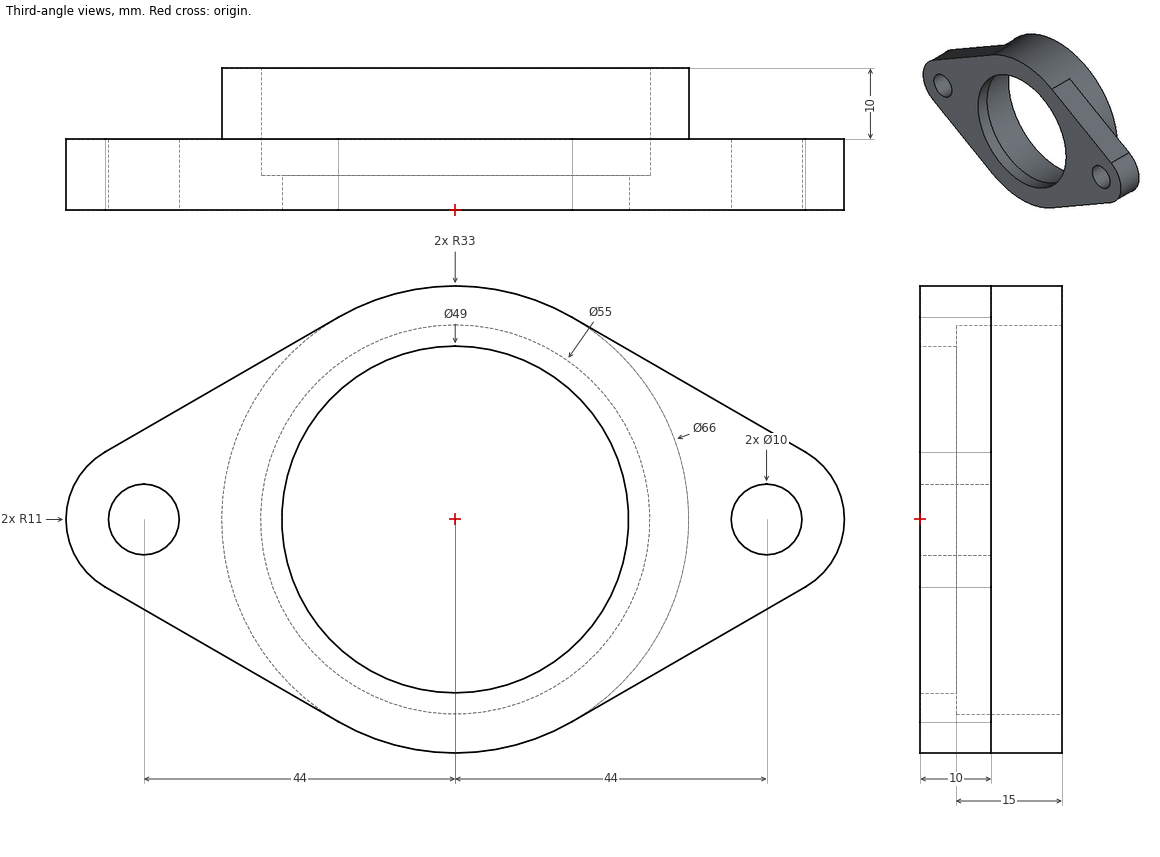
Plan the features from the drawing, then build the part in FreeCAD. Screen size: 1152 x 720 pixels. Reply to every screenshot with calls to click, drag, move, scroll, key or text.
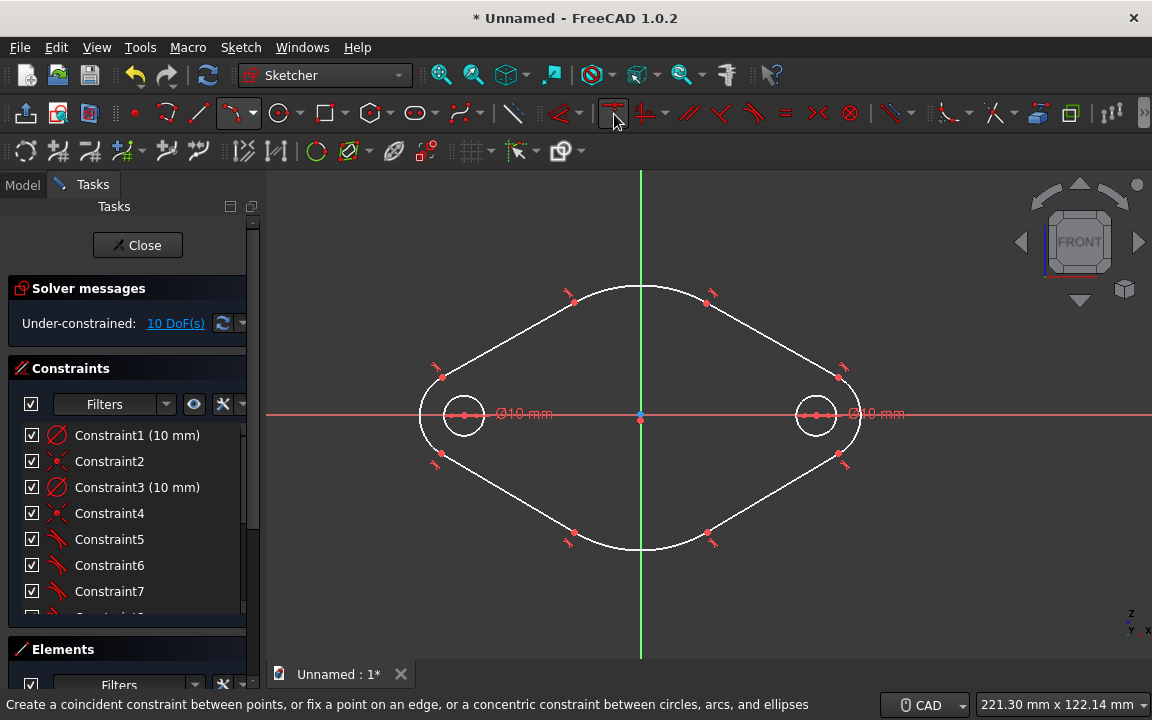
scroll(641, 417, up, 4)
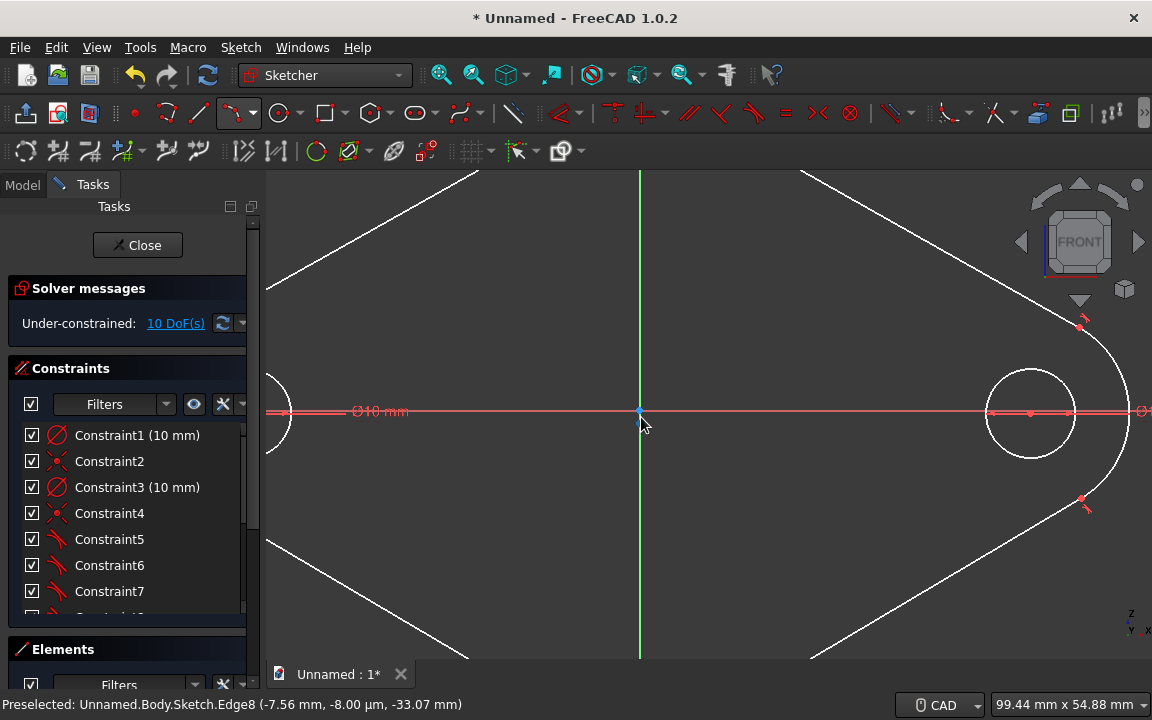
drag(630, 401, 650, 434)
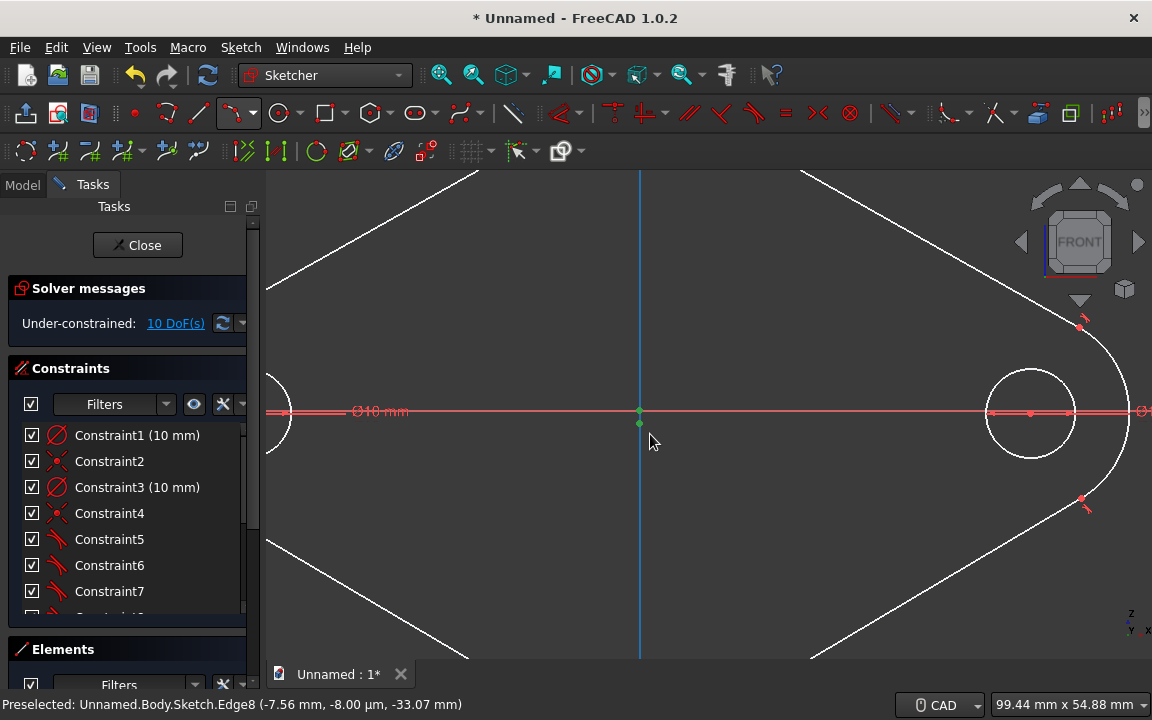
click(614, 114)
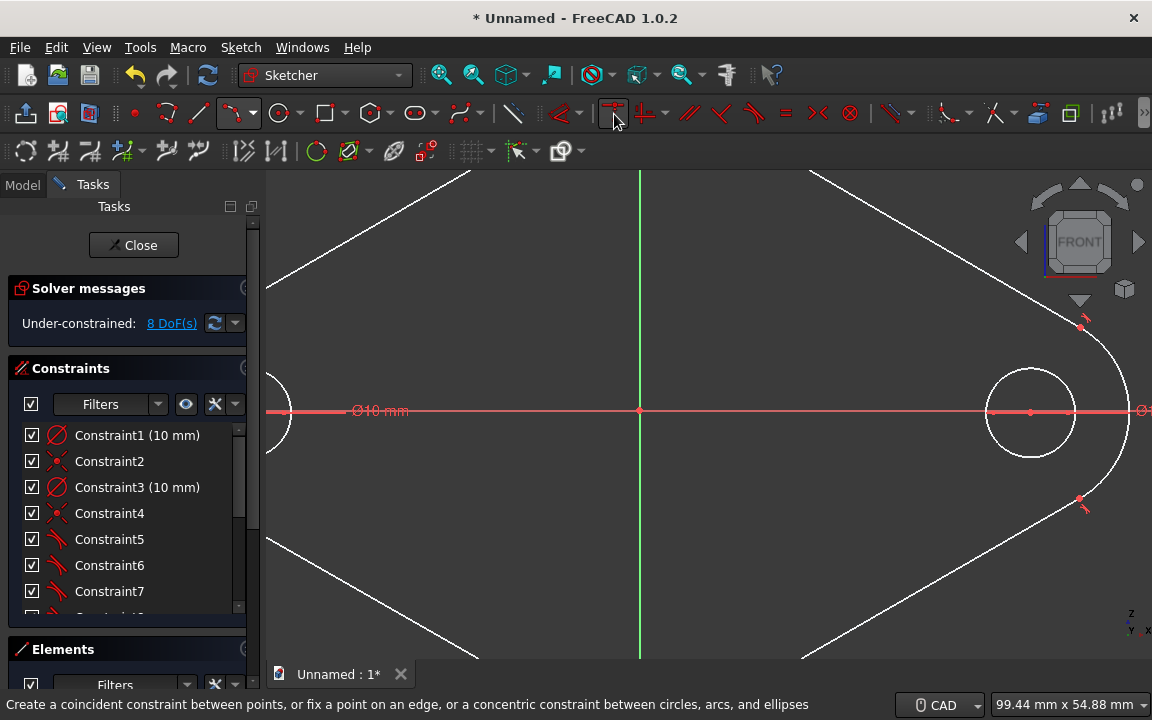
scroll(641, 419, down, 3)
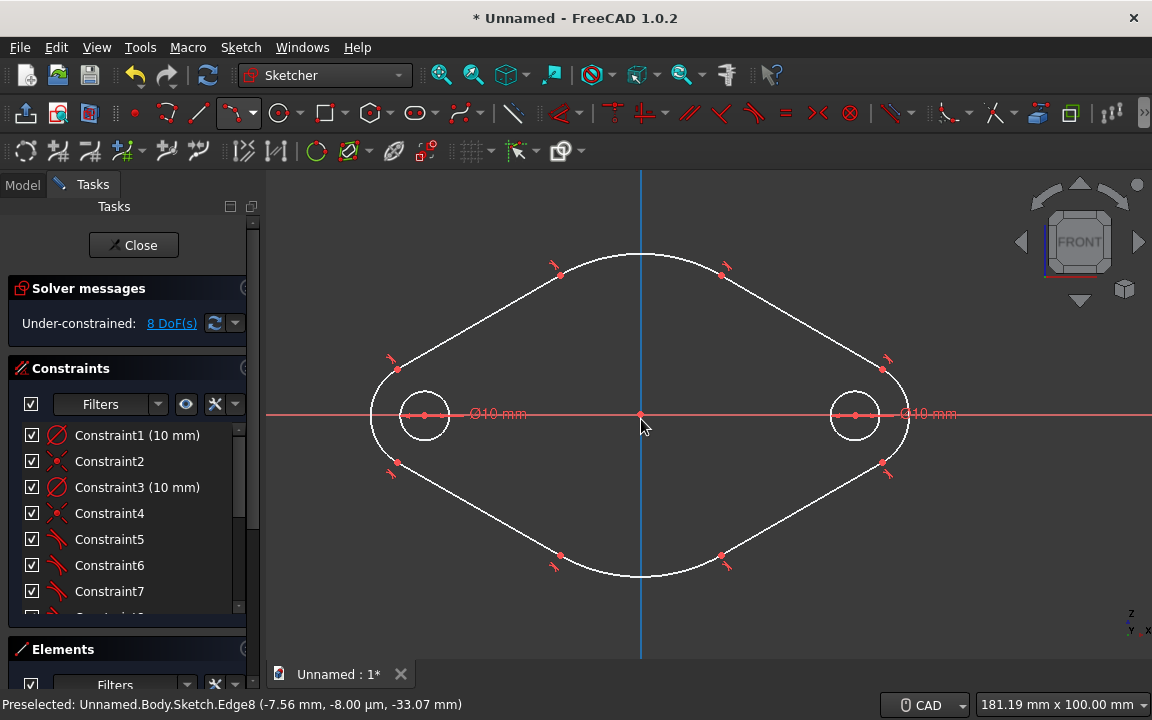
click(375, 394)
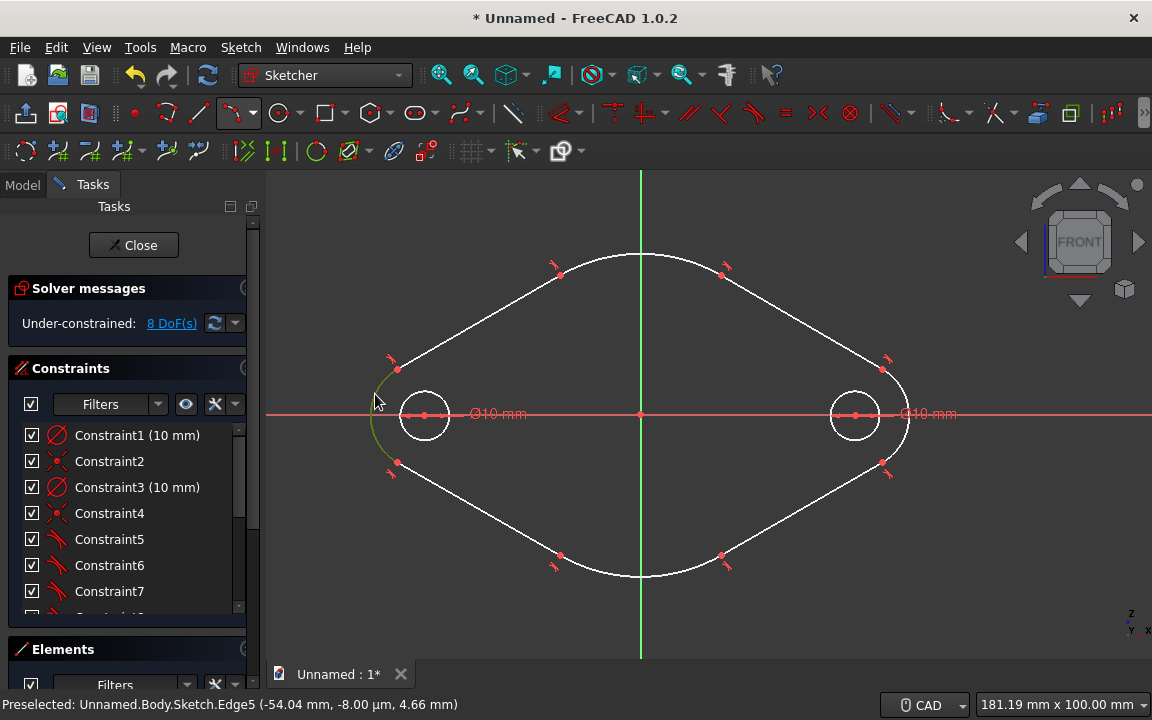
click(904, 438)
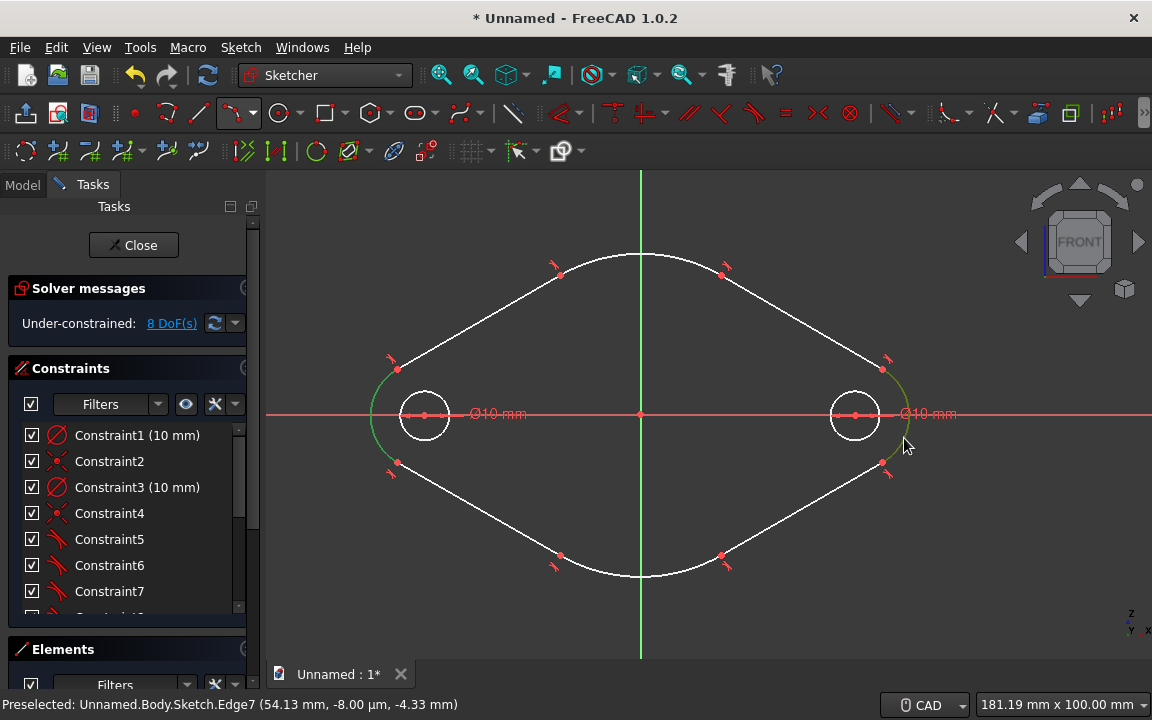
click(786, 114)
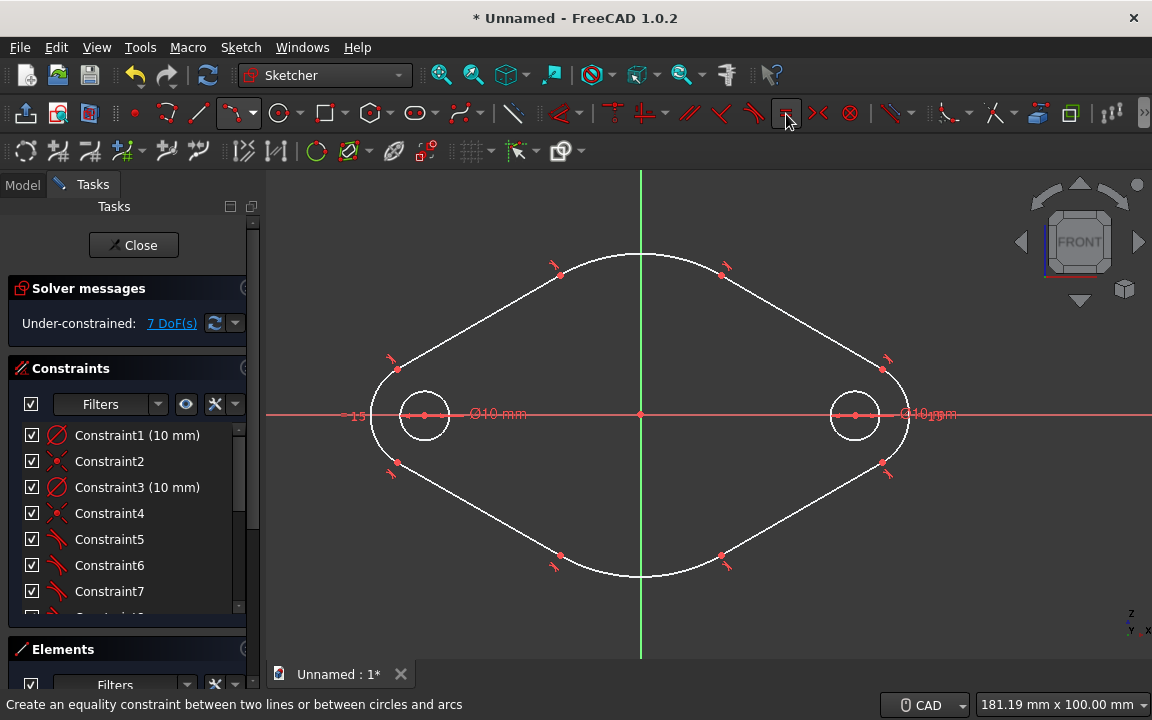
click(674, 257)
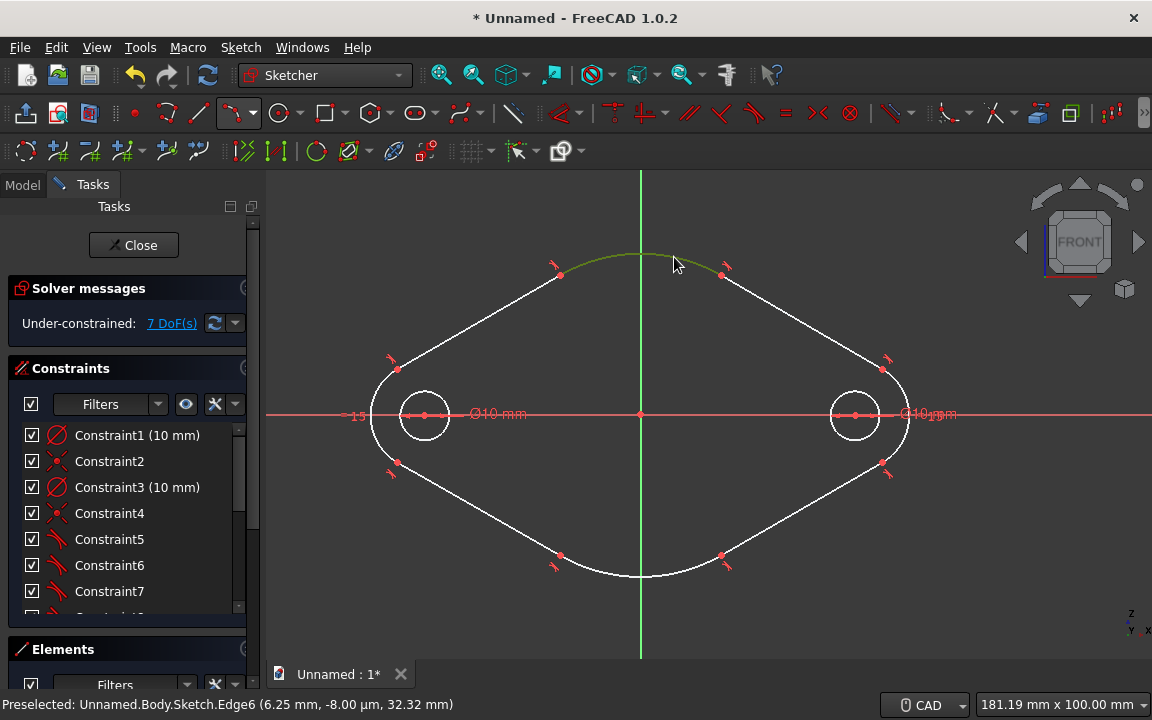
click(607, 573)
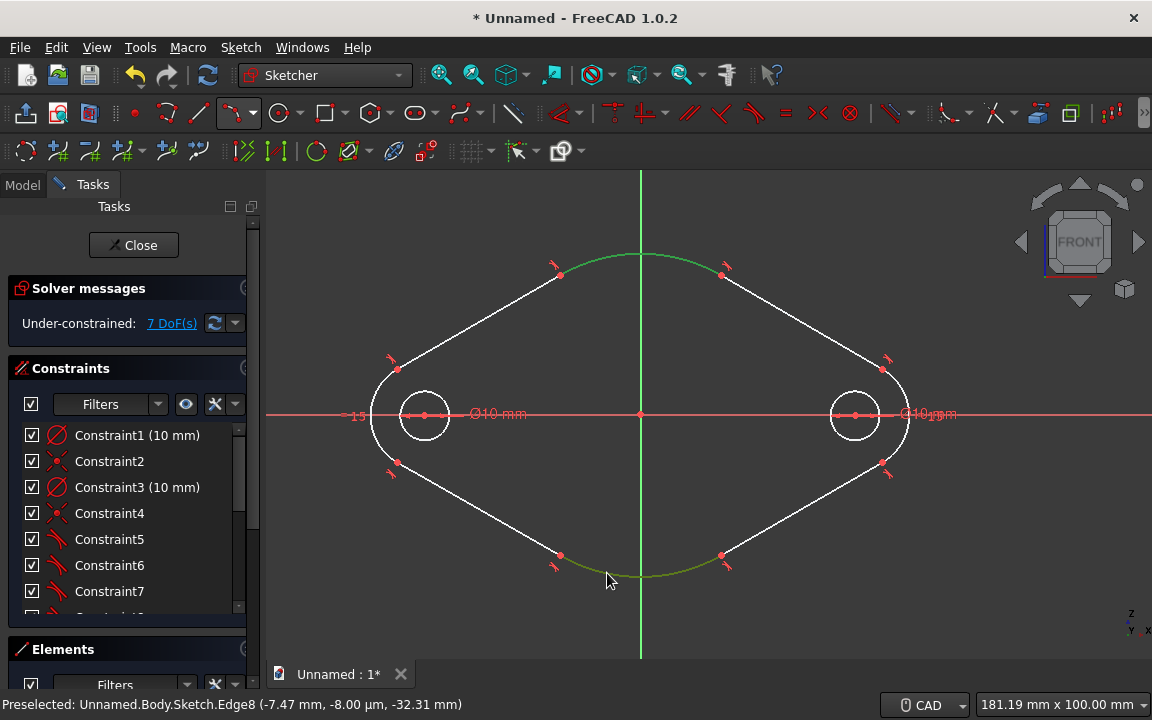
click(786, 114)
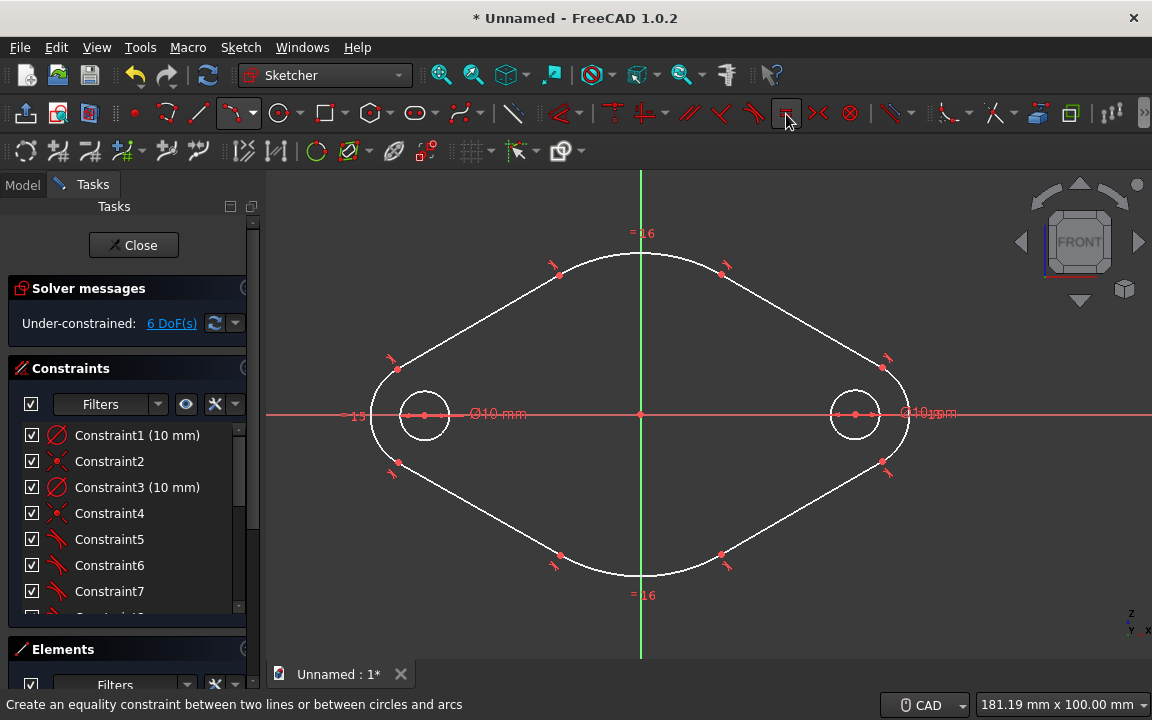
click(425, 416)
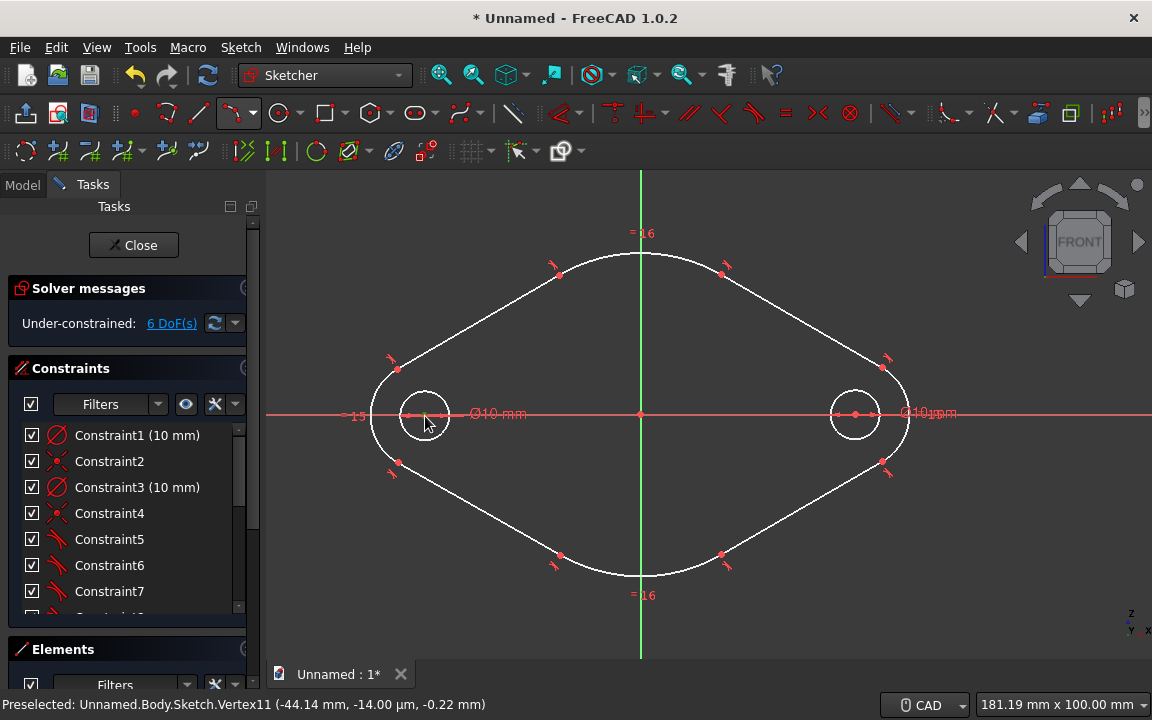
click(542, 415)